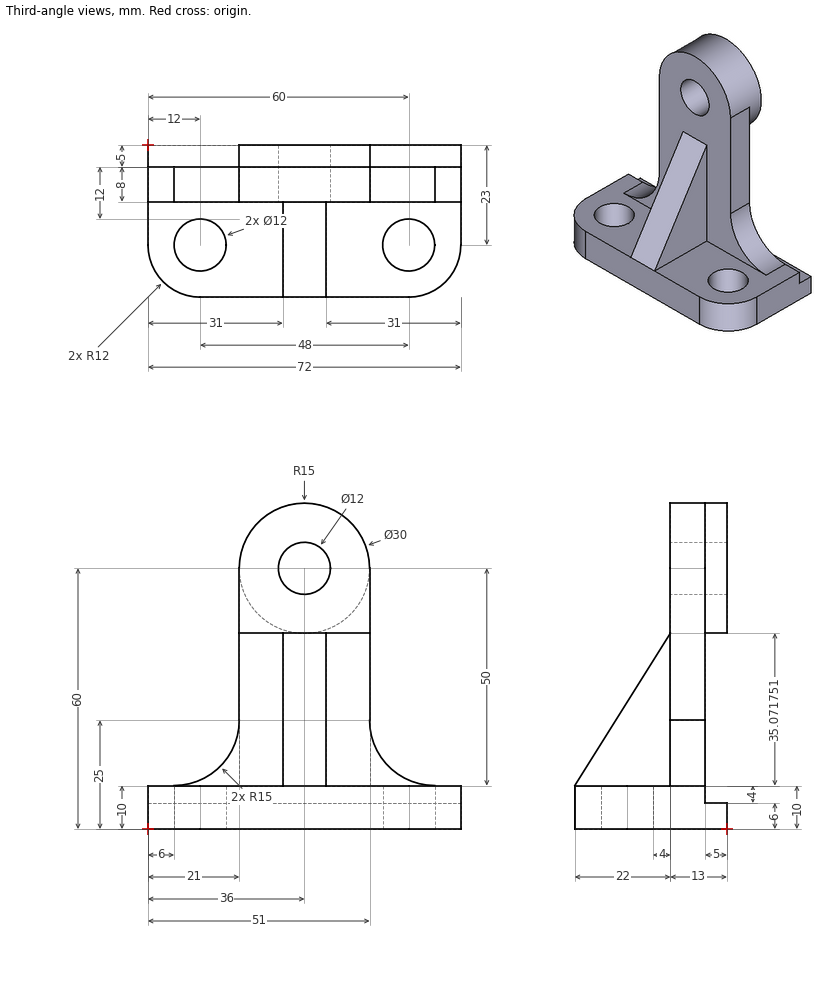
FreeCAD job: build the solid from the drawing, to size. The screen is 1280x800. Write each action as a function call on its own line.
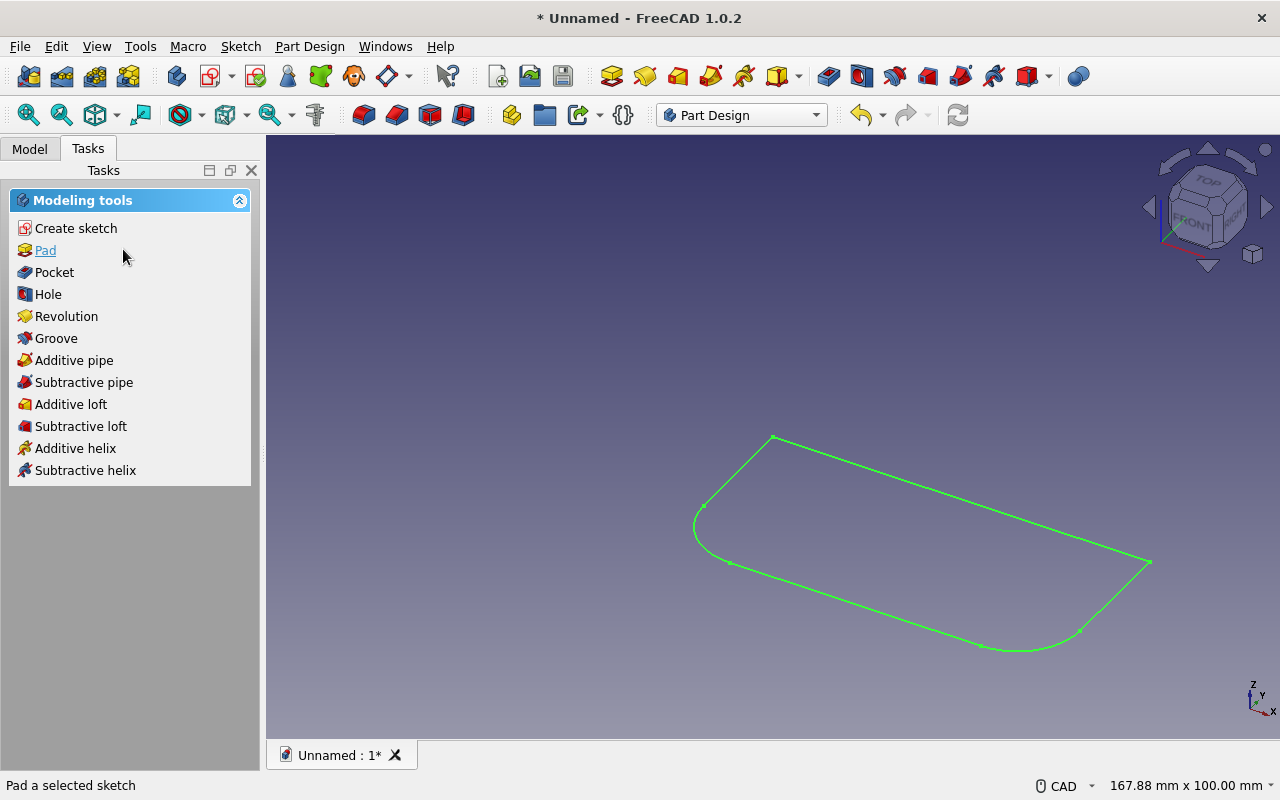
click(612, 76)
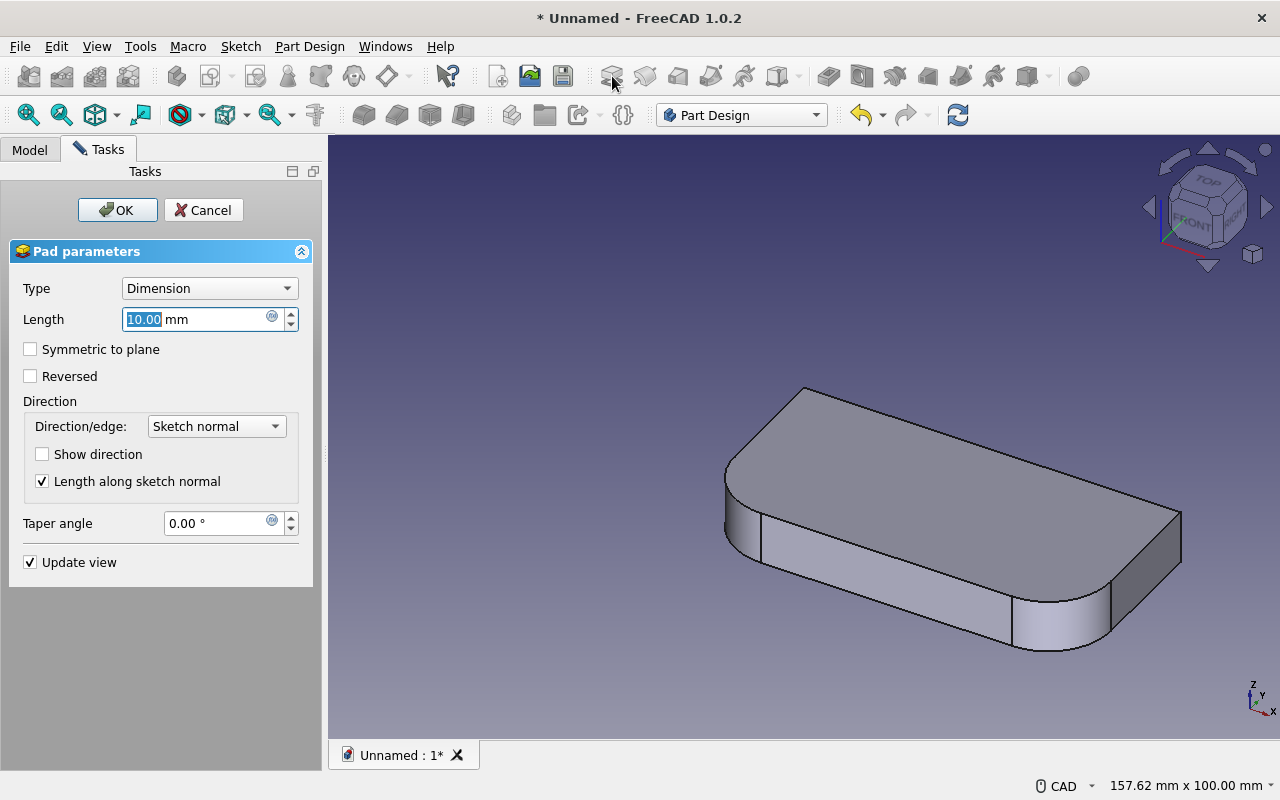
text(10)
key(Tab)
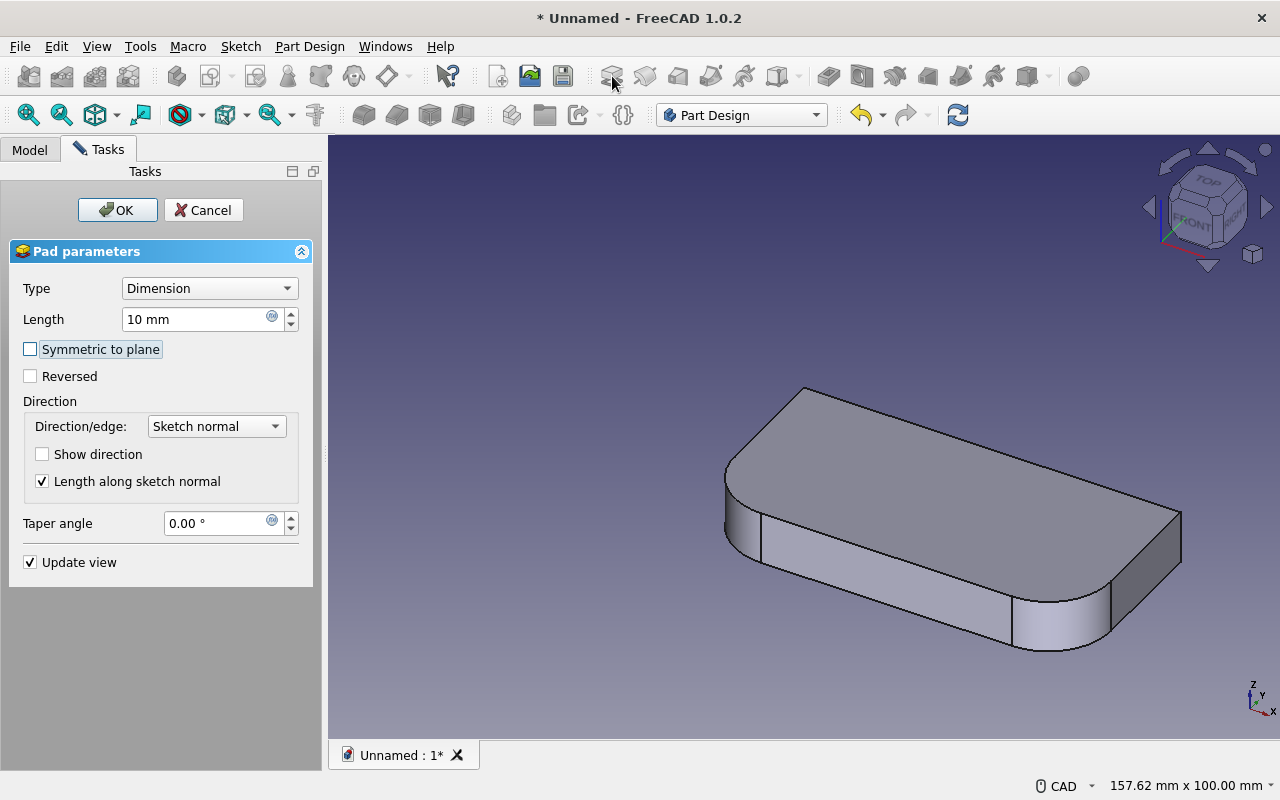
click(118, 210)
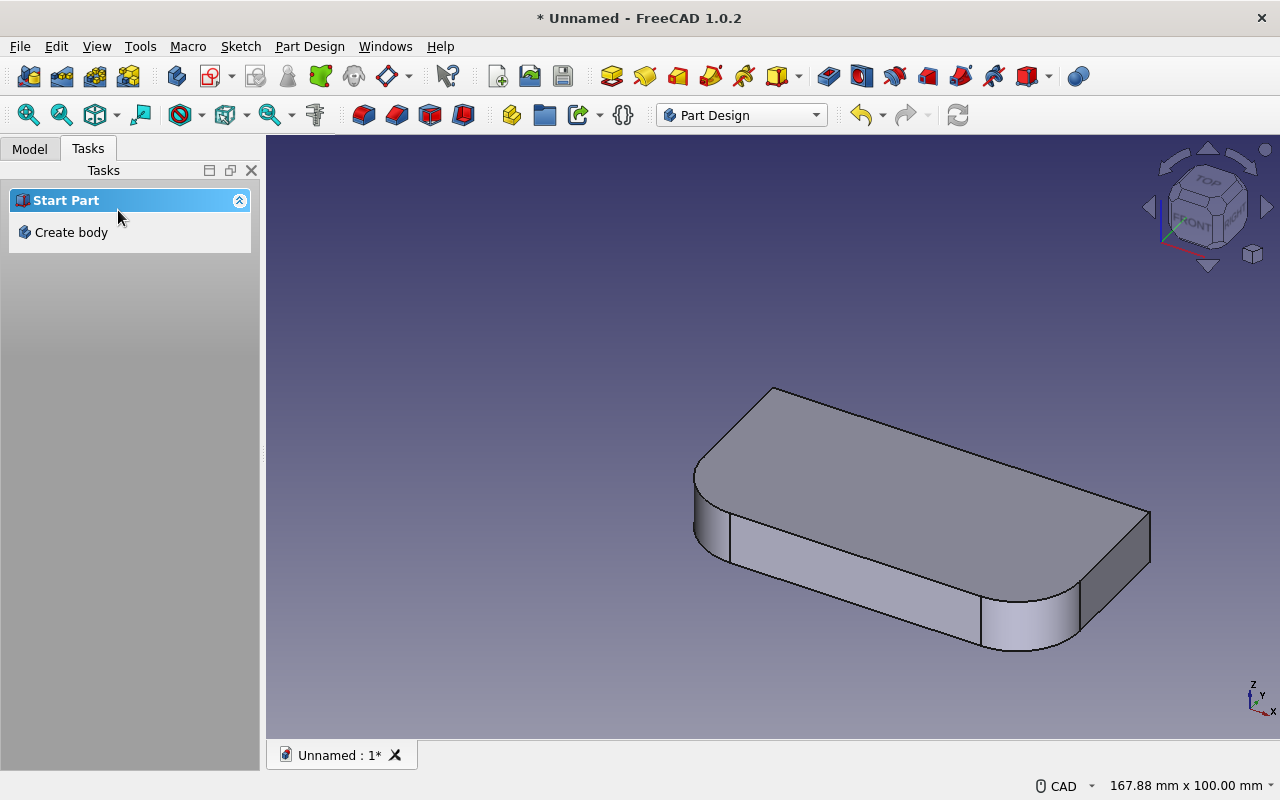
click(1125, 561)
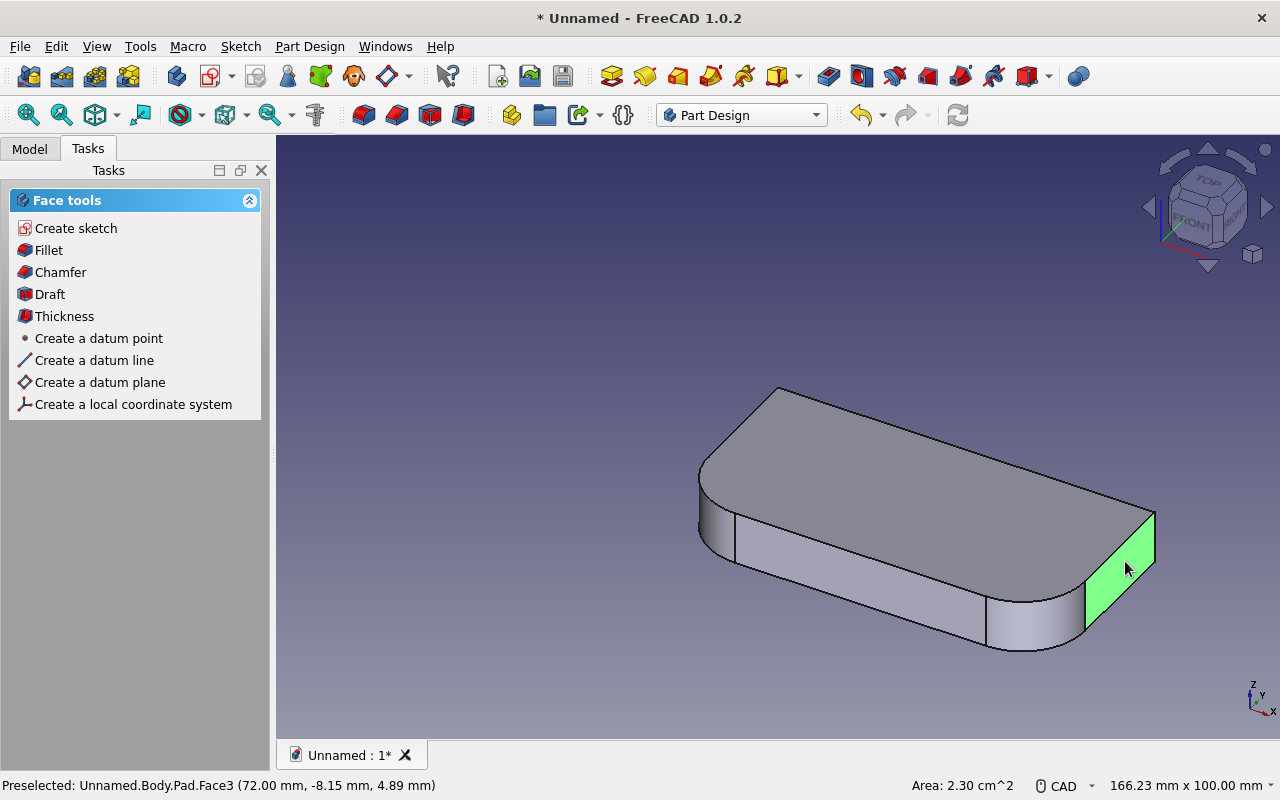
click(210, 76)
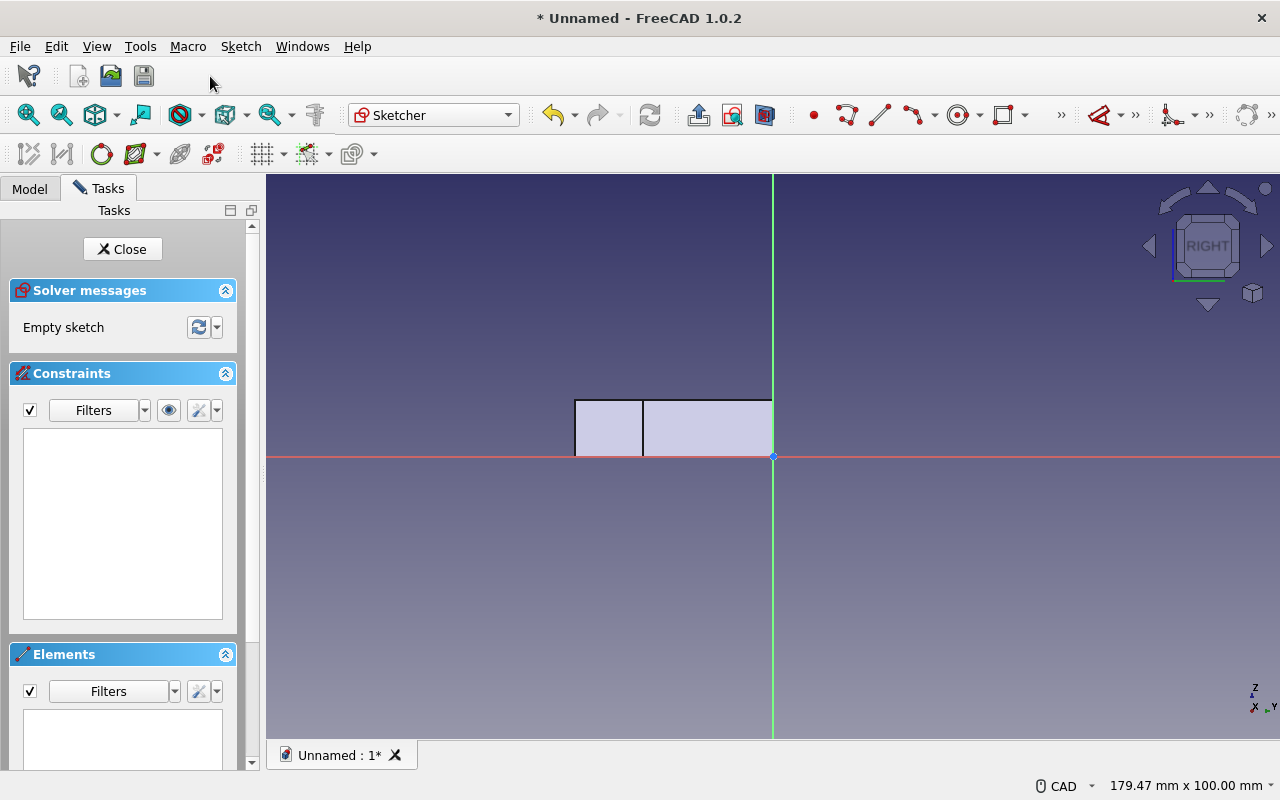
scroll(770, 423, up, 9)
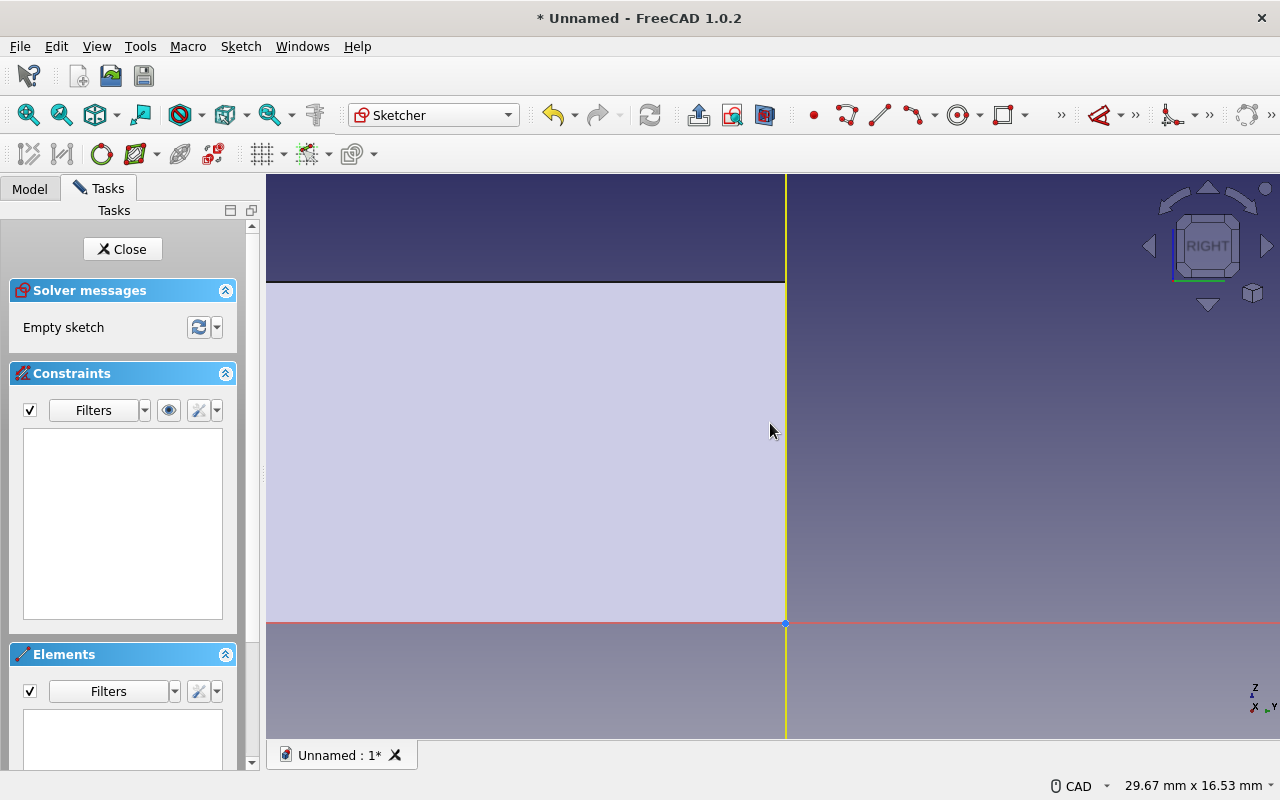
key(g)
key(r)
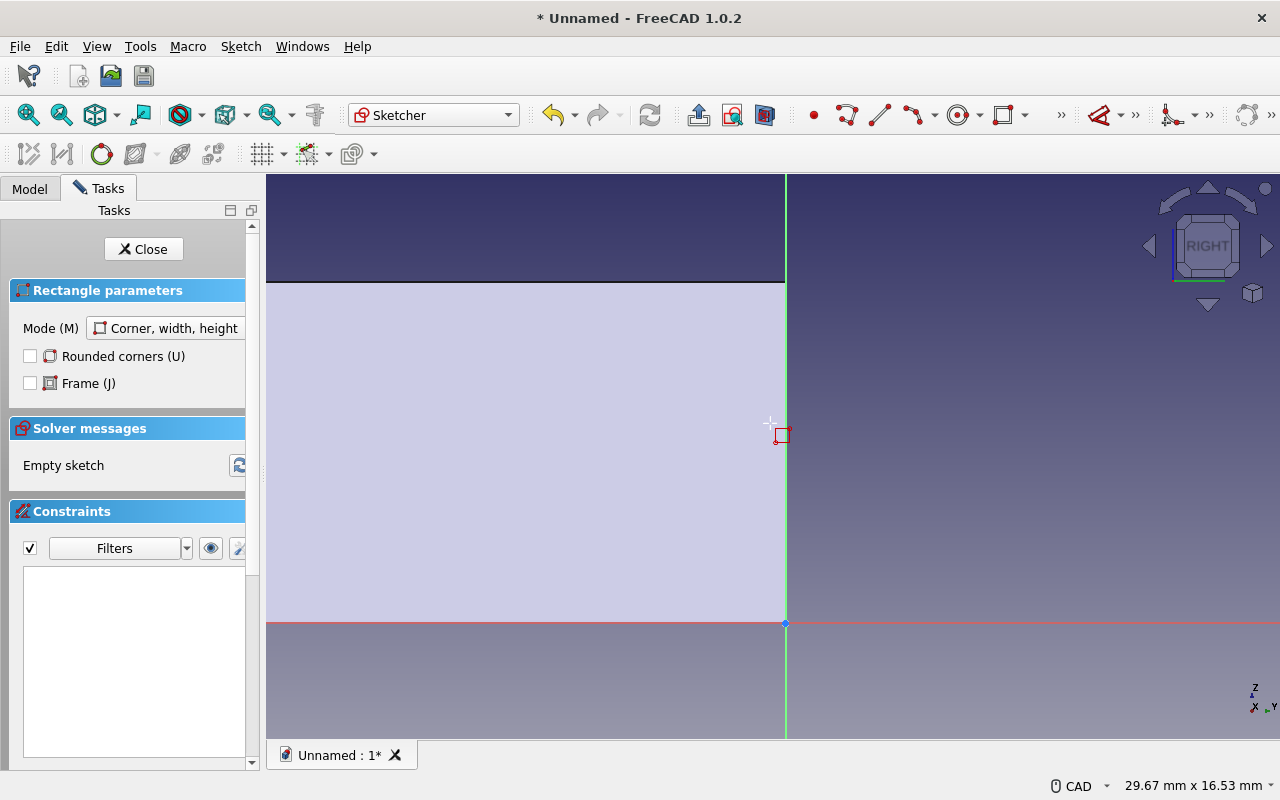
click(615, 282)
click(786, 418)
key(Escape)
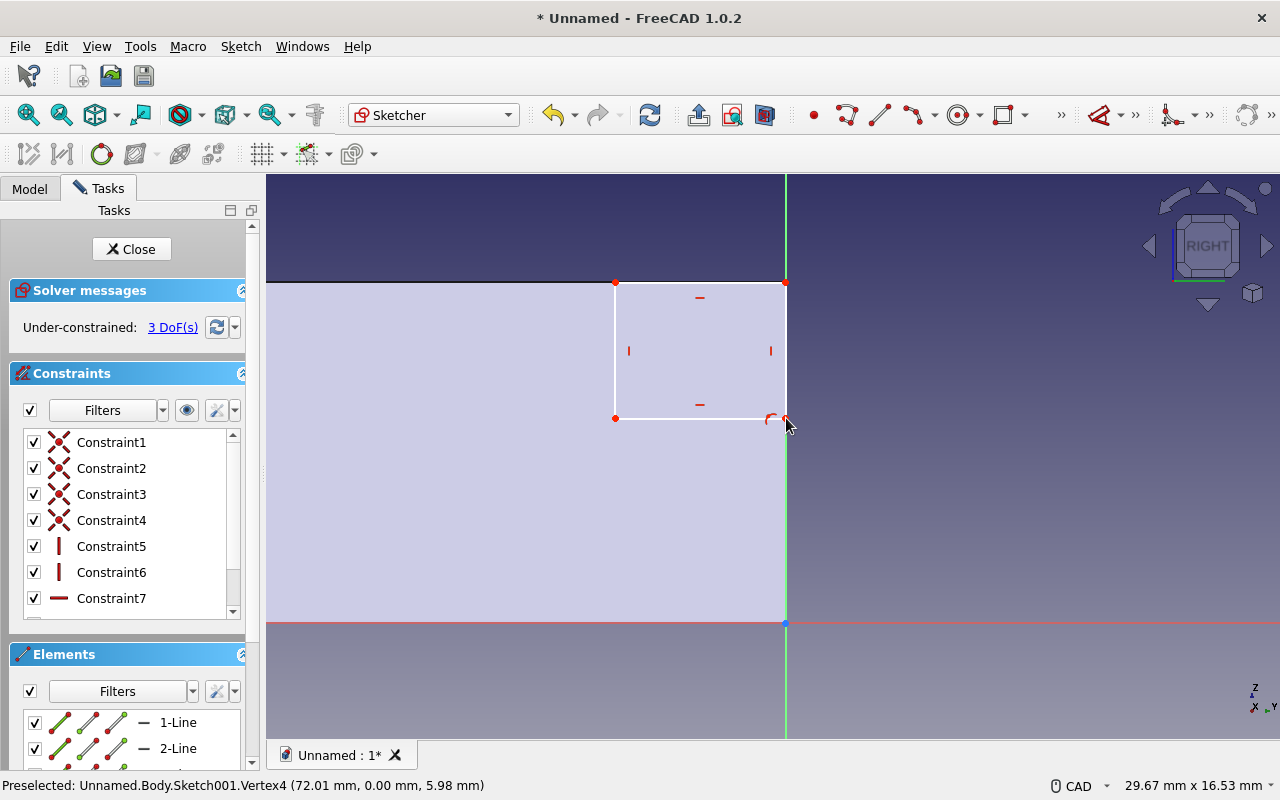
click(1098, 116)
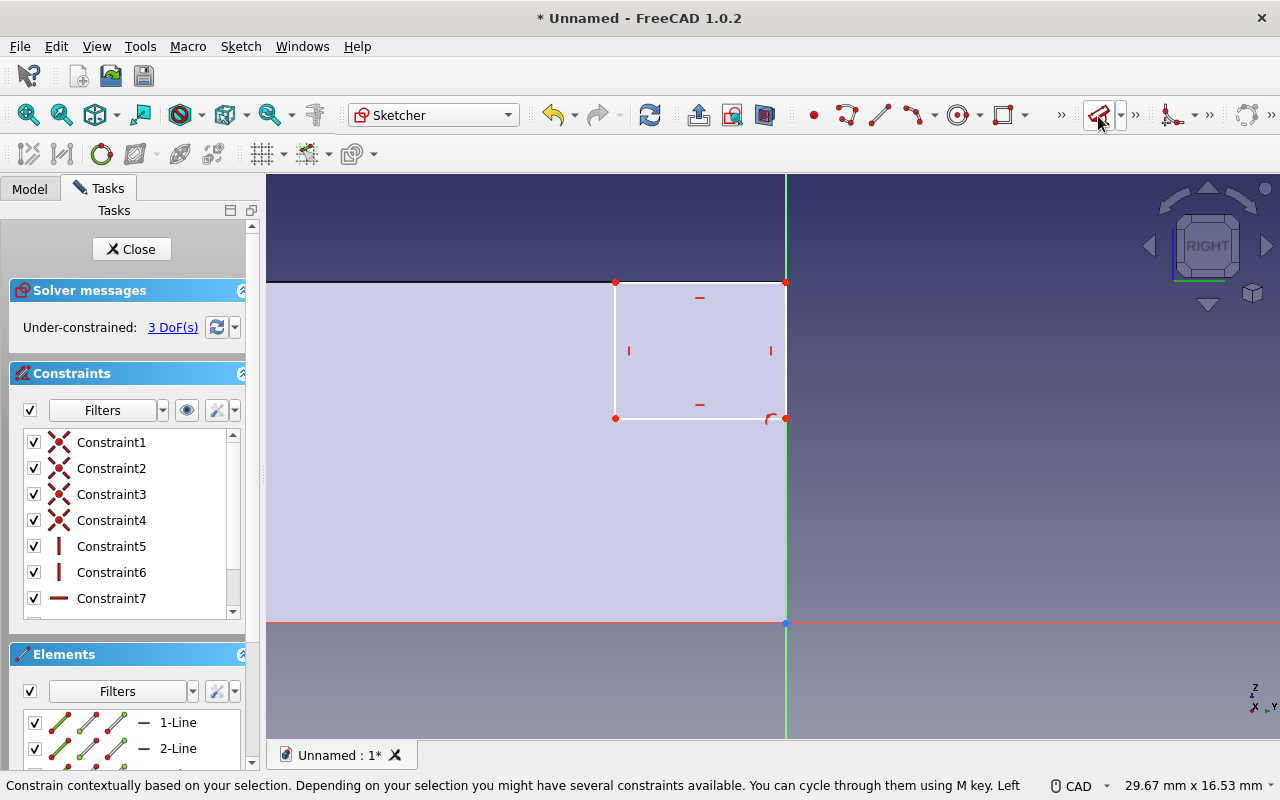
click(615, 324)
click(581, 351)